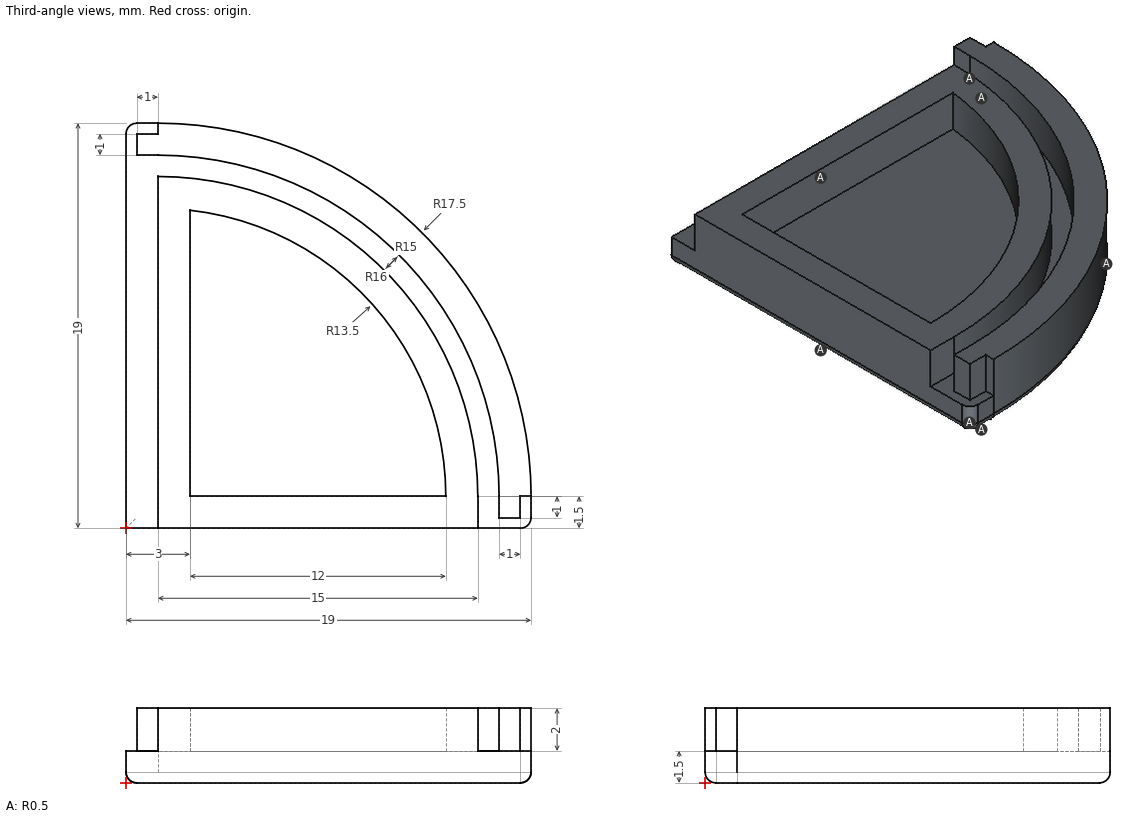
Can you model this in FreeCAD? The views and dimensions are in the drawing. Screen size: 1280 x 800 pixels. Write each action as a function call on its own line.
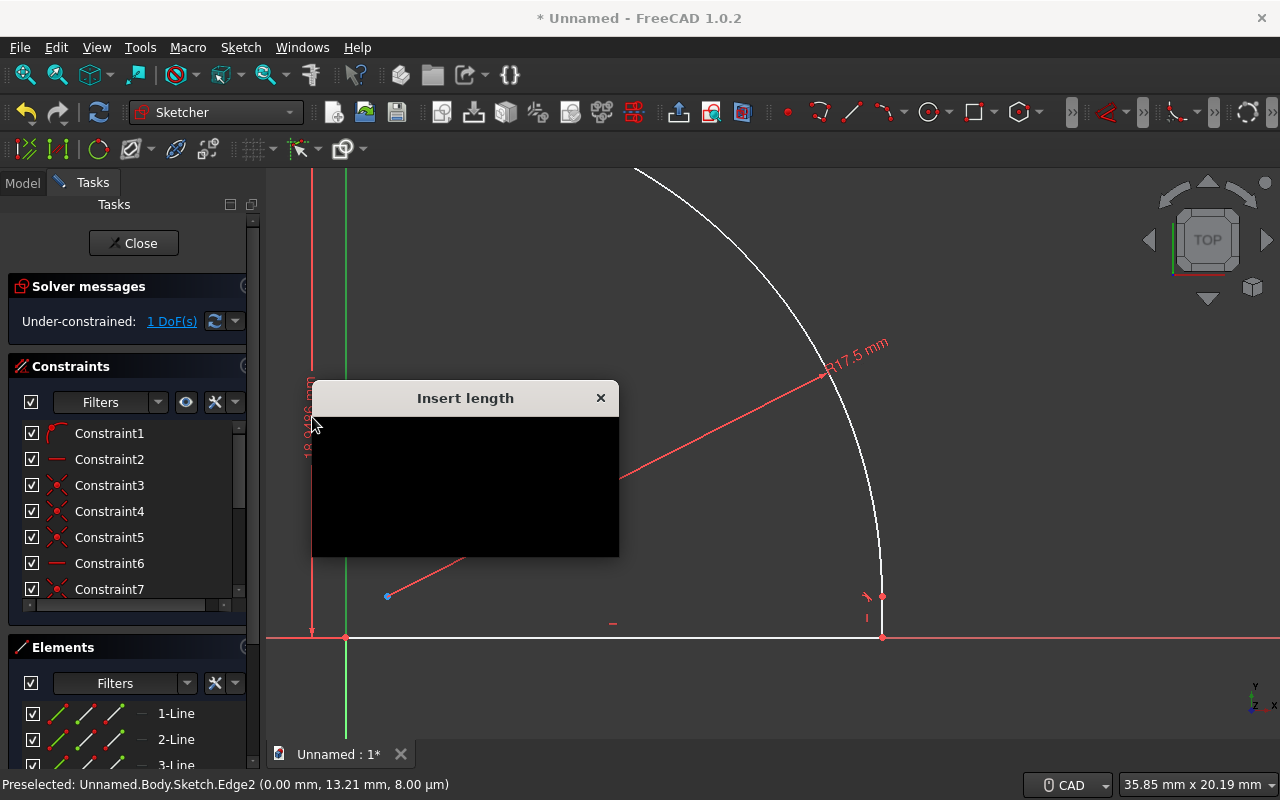
text(19)
key(Return)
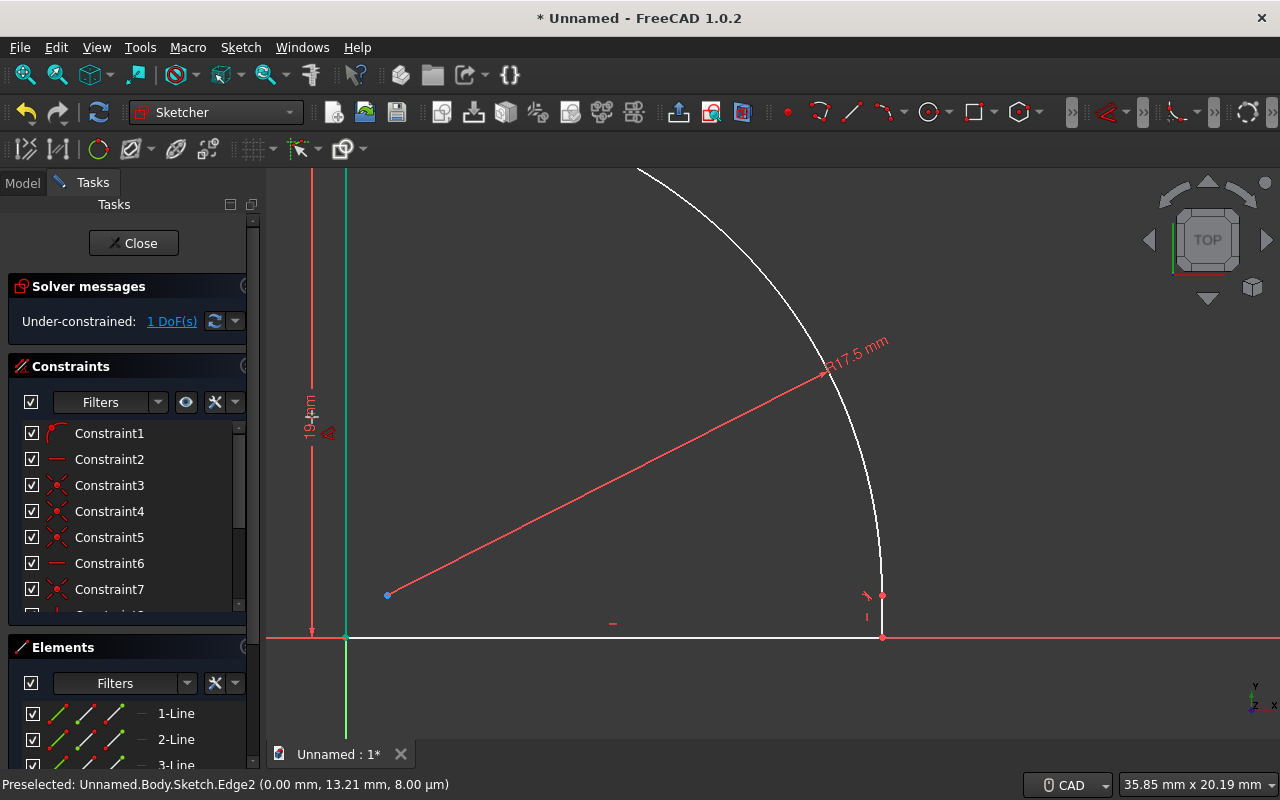
click(507, 638)
click(614, 672)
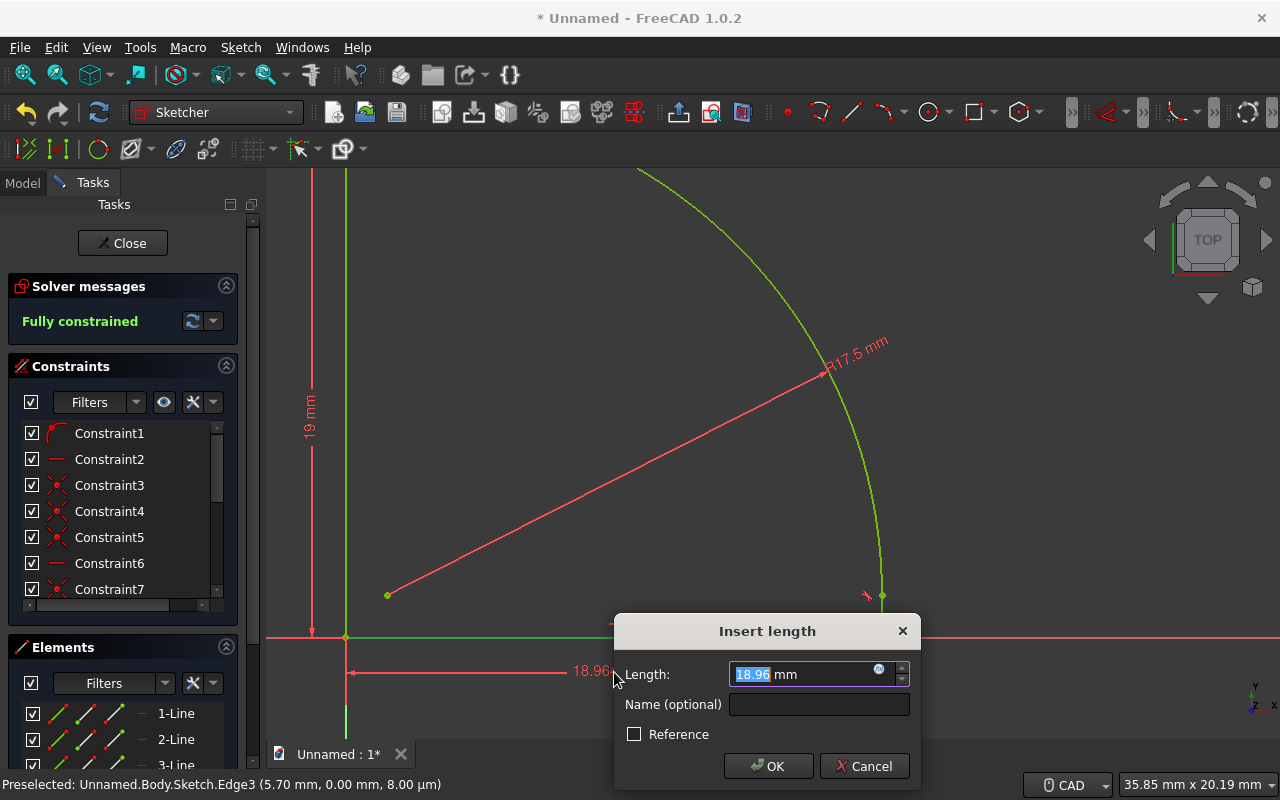
text(19)
key(Return)
key(Escape)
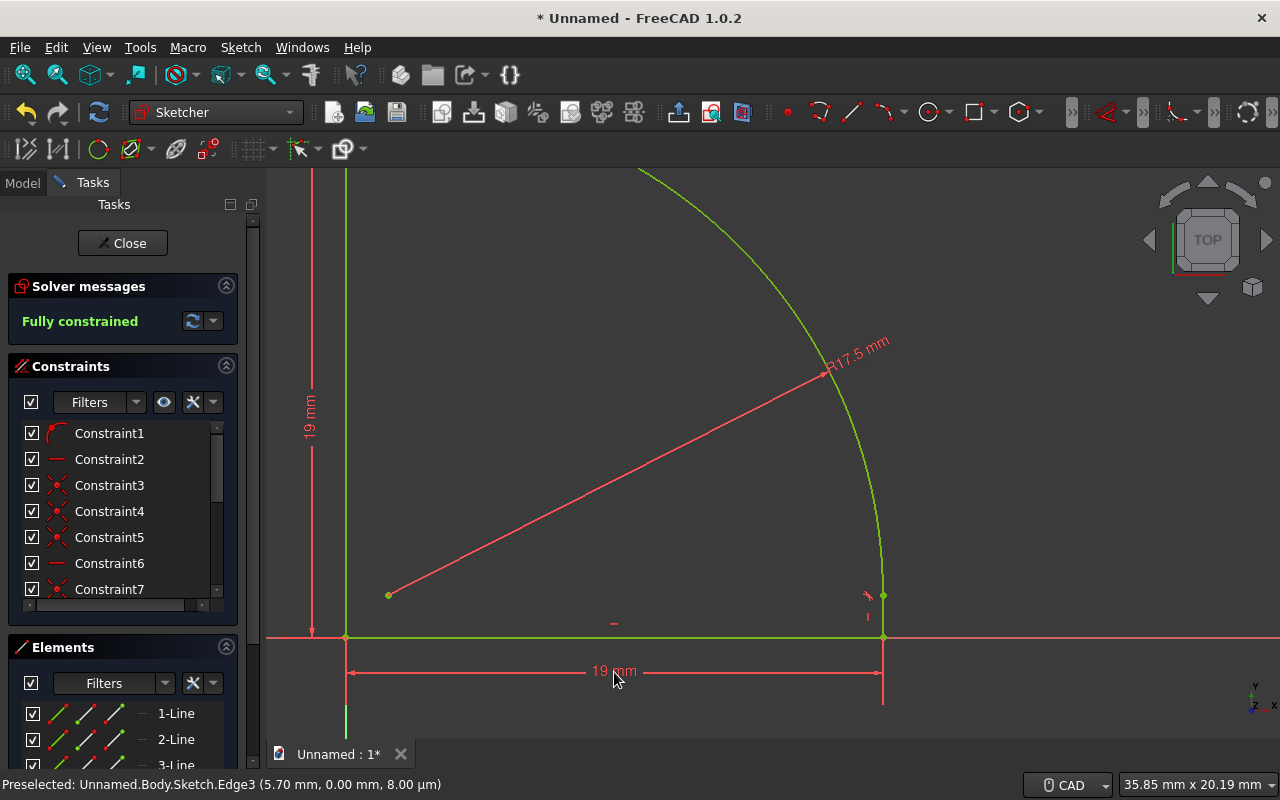
click(123, 243)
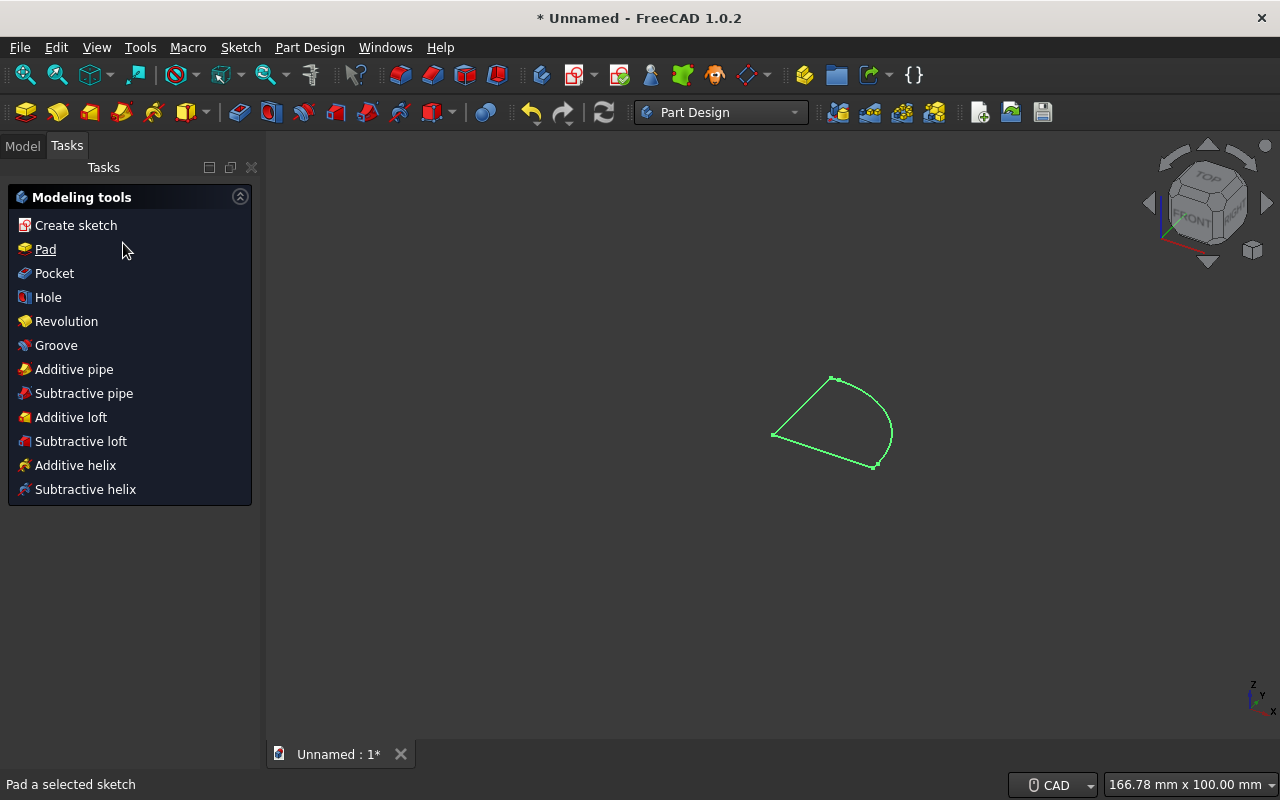
click(26, 112)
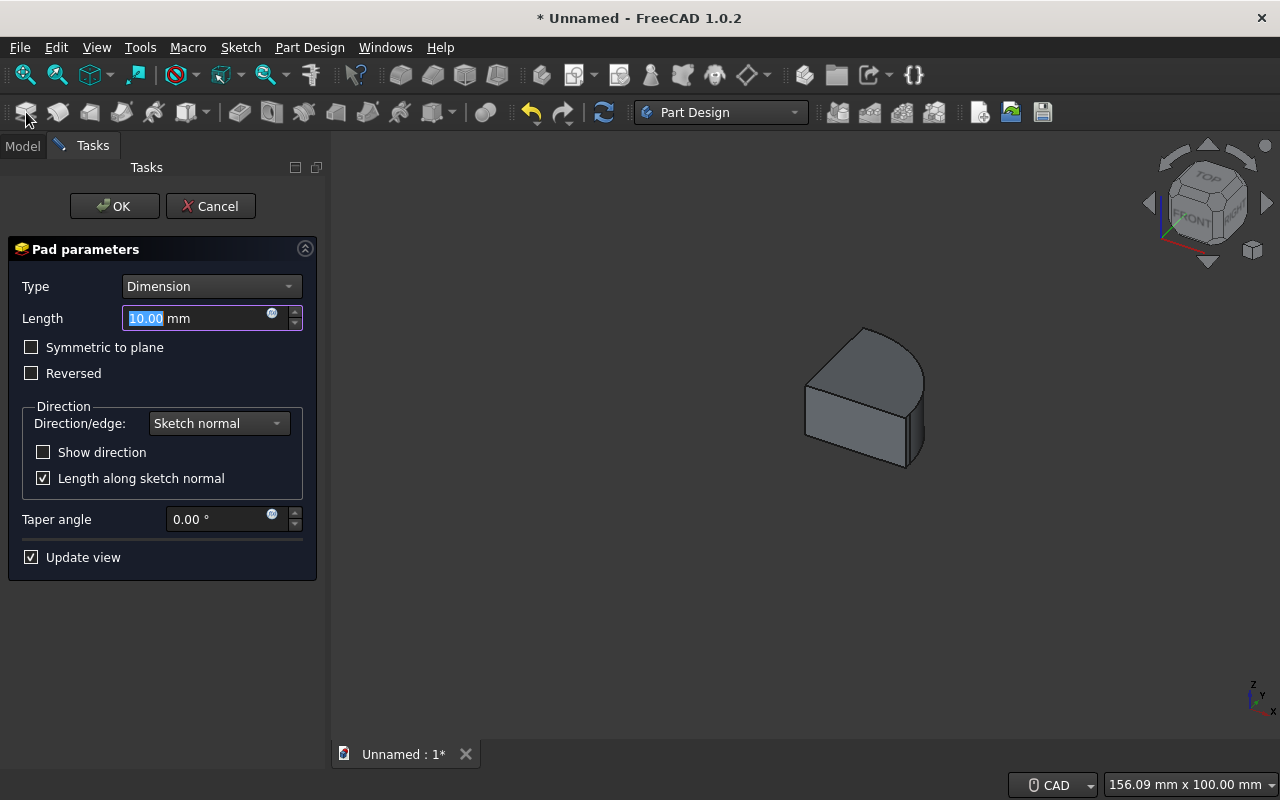
text(1.5)
key(Tab)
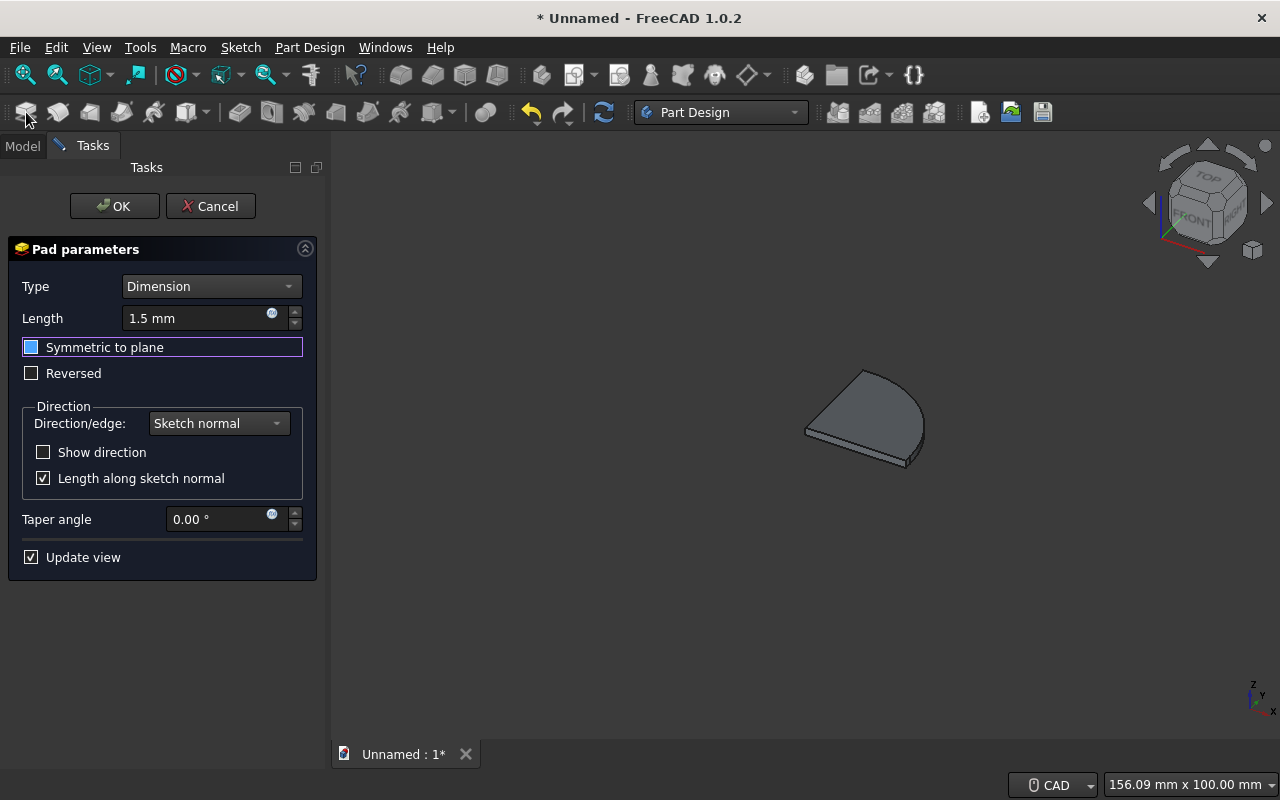
click(115, 206)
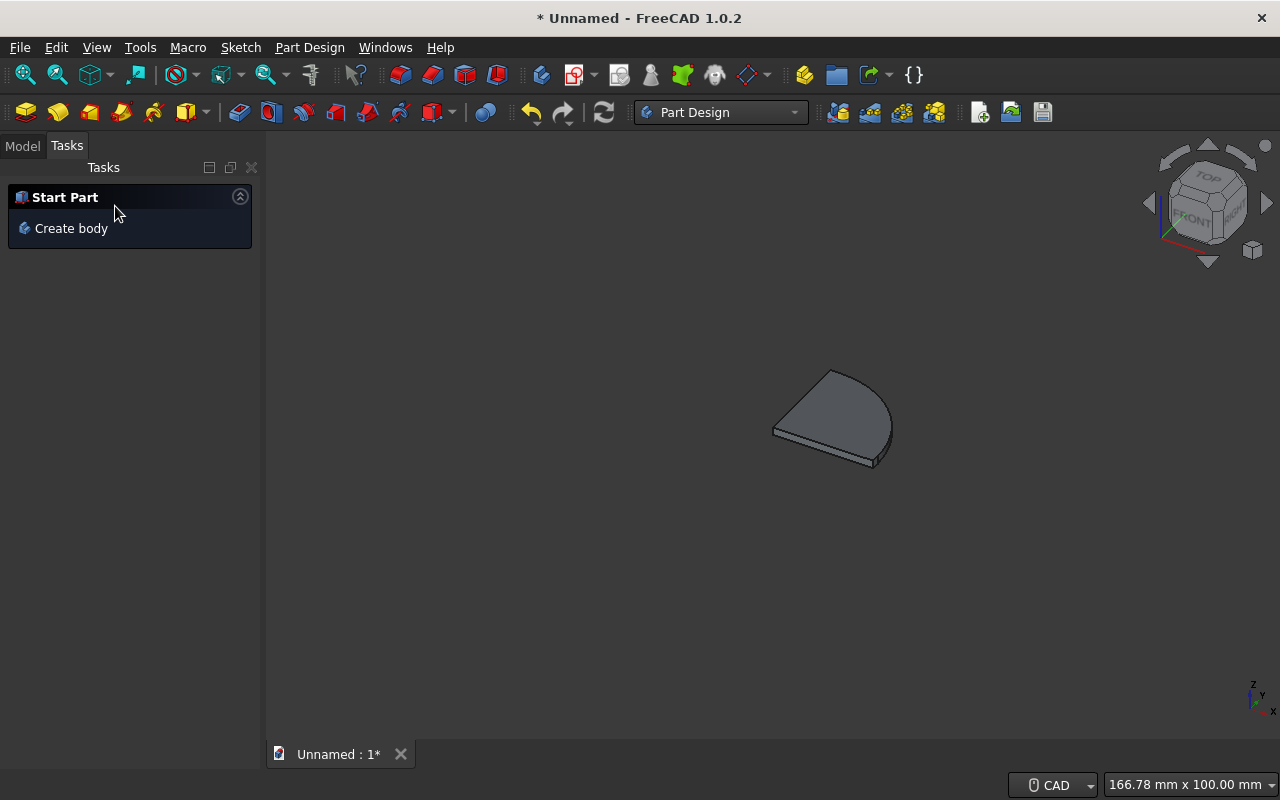
key(v)
key(f)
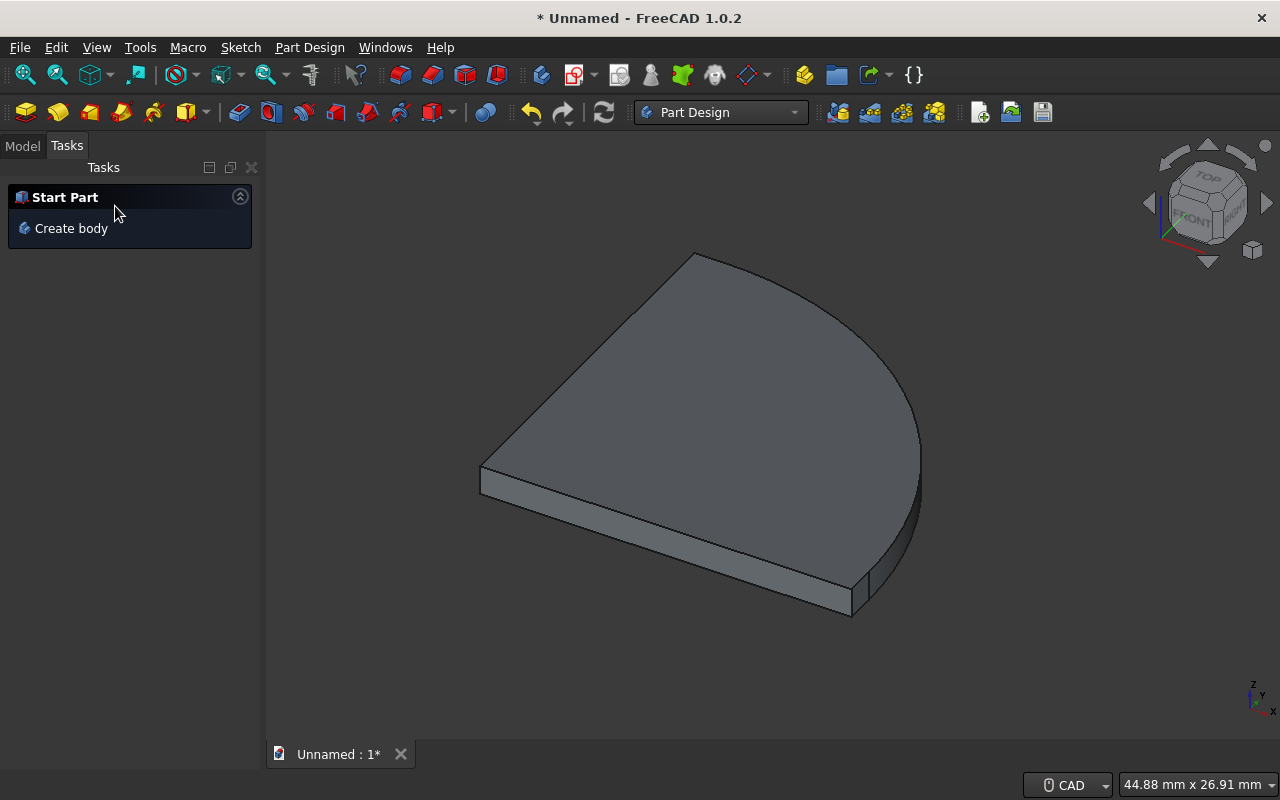
click(742, 451)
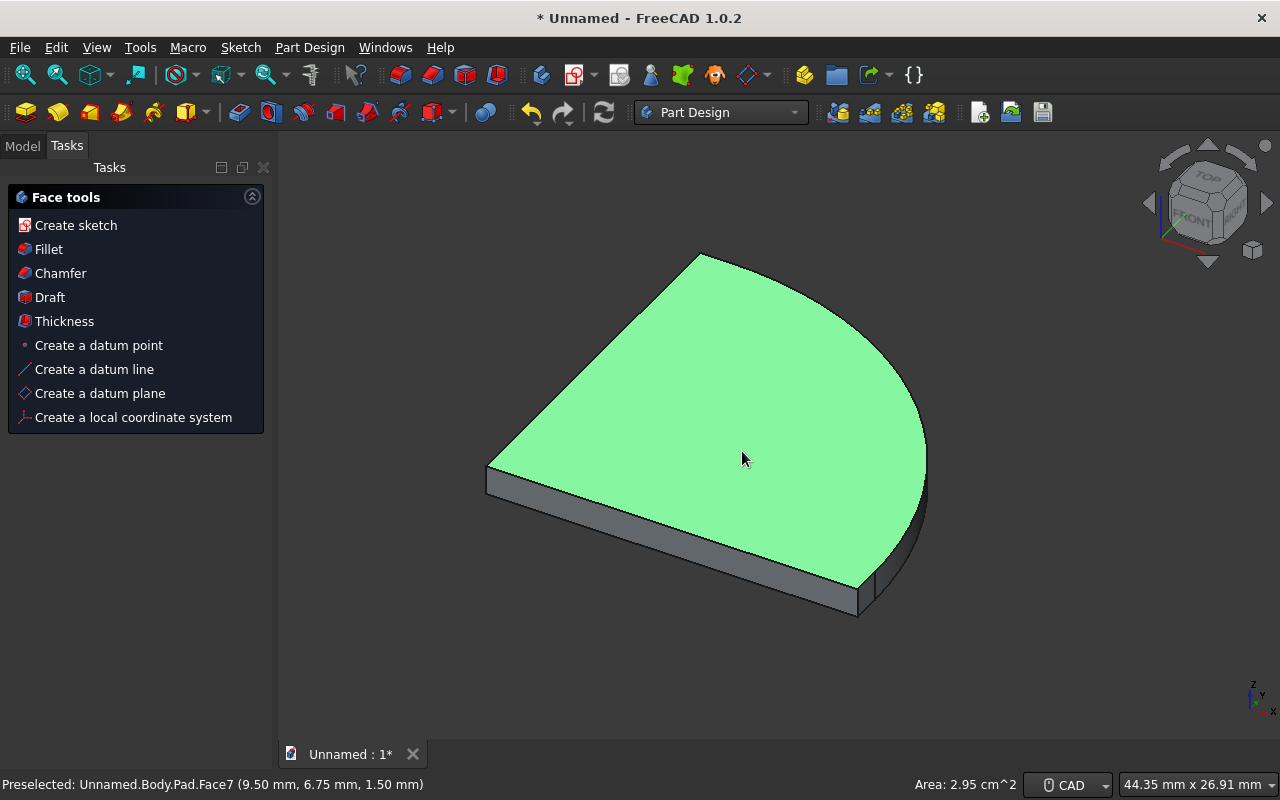
click(574, 76)